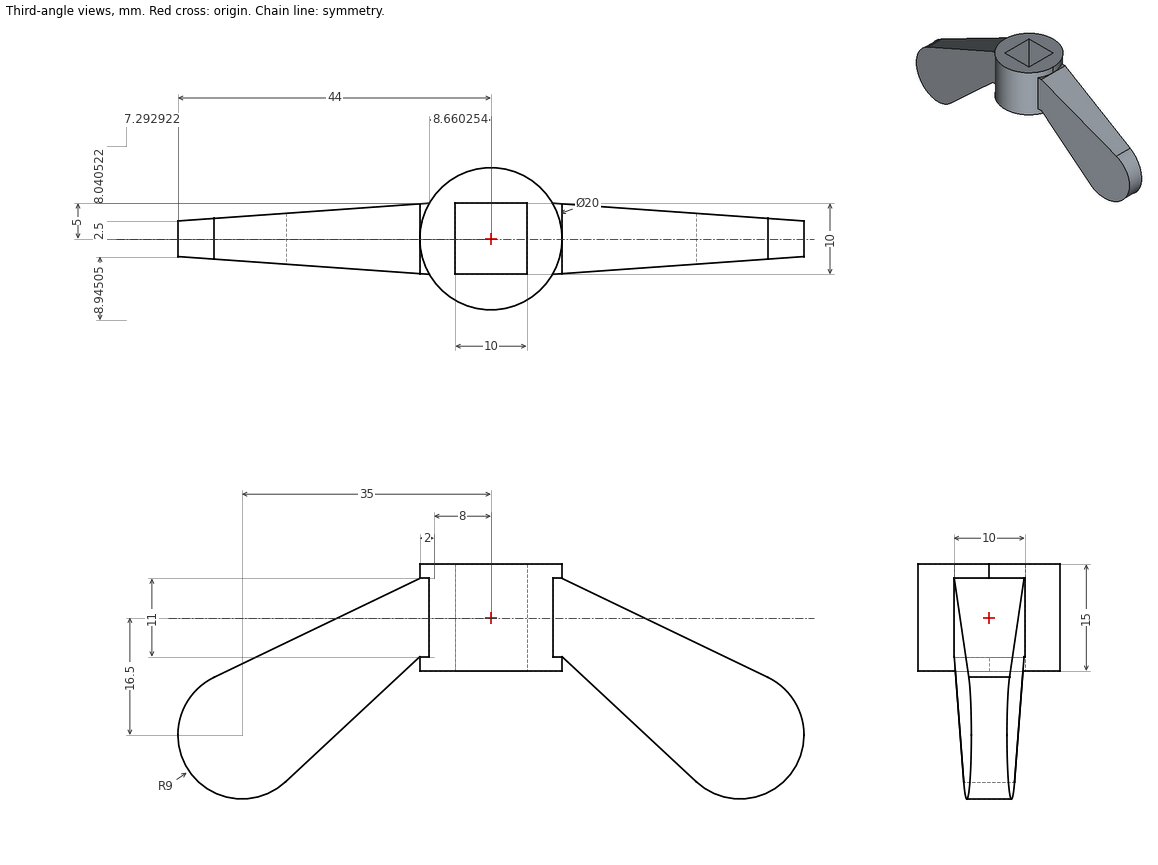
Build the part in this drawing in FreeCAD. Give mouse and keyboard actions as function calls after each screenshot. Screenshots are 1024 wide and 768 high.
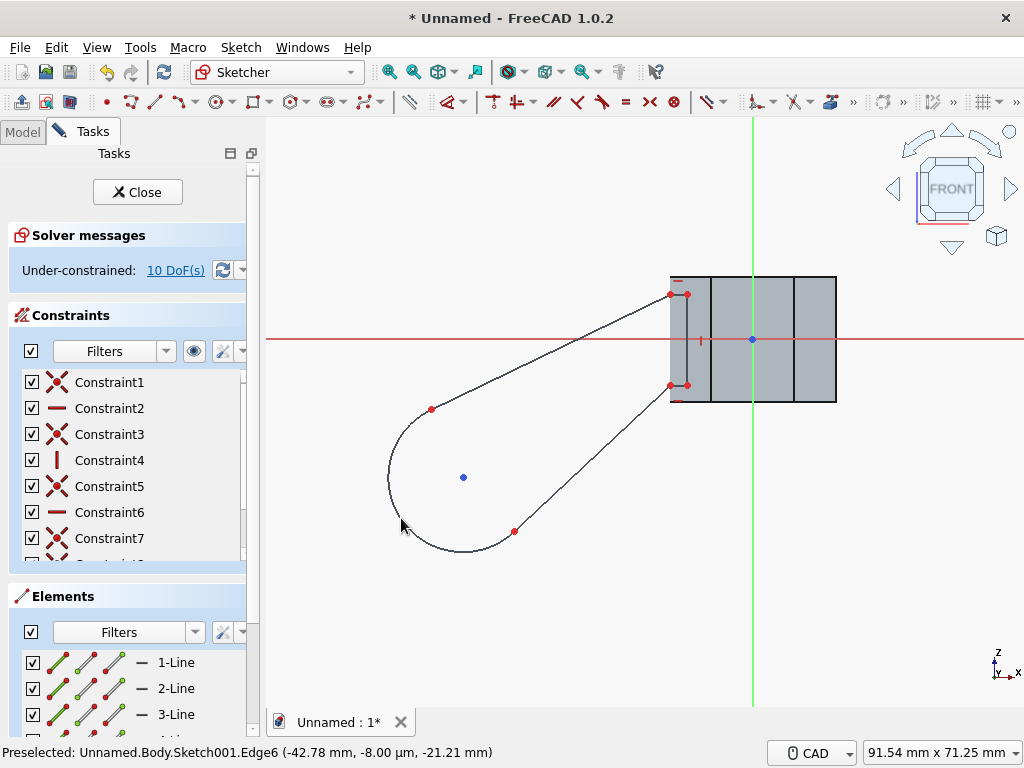
click(503, 375)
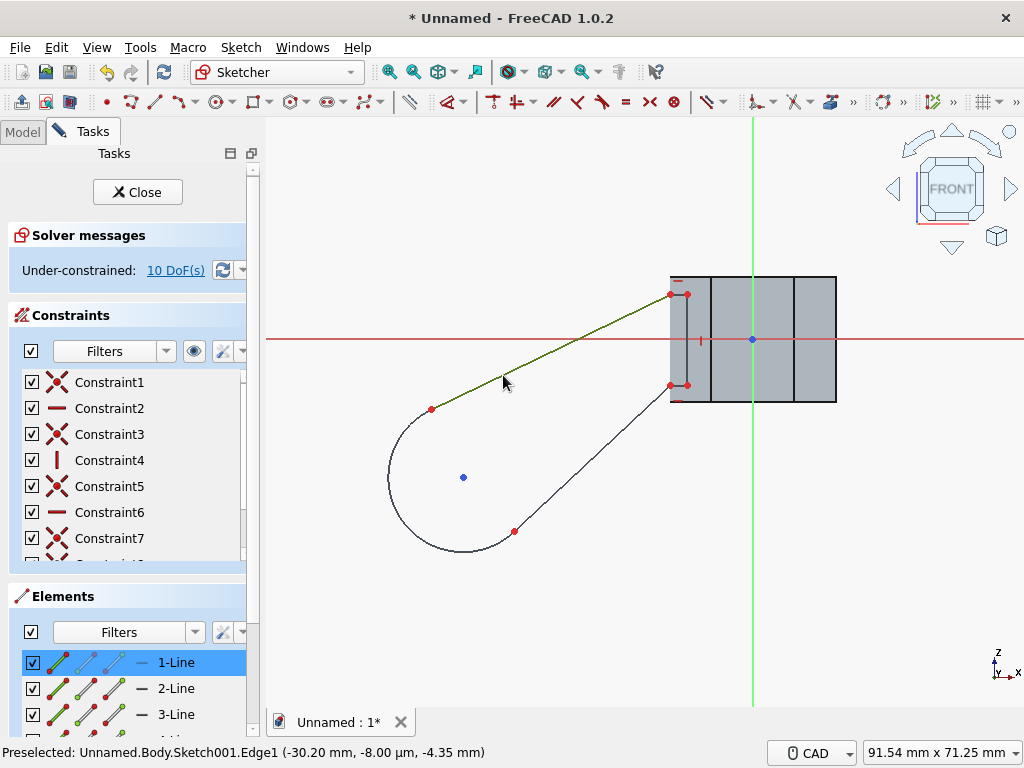
click(389, 471)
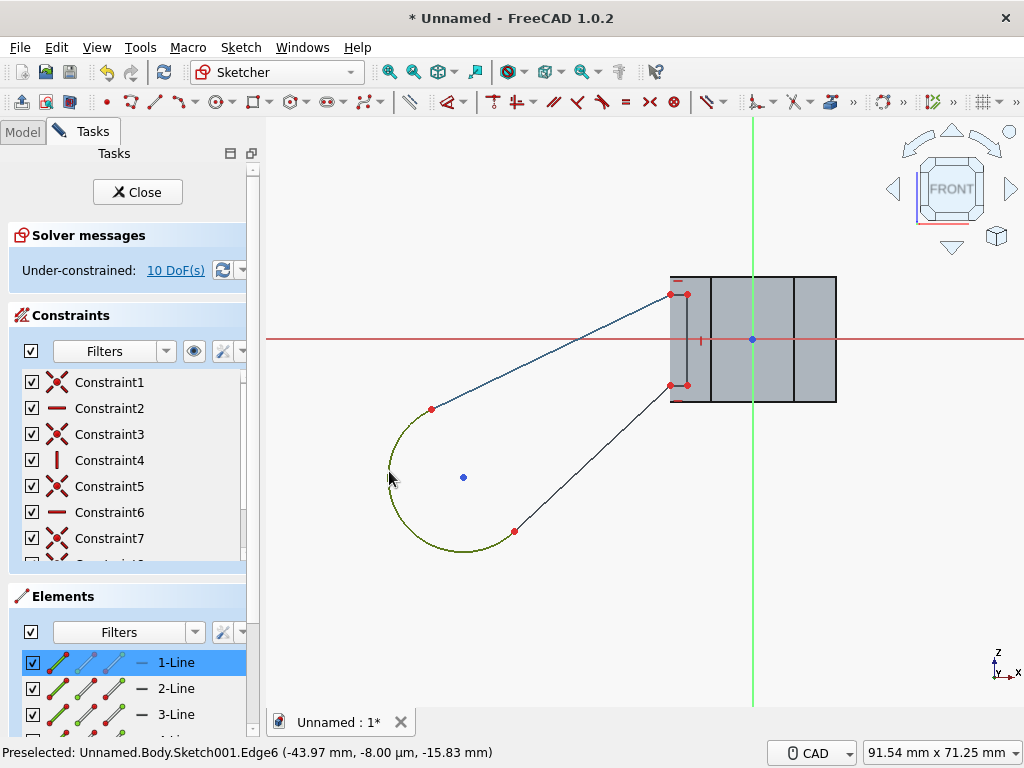
click(602, 102)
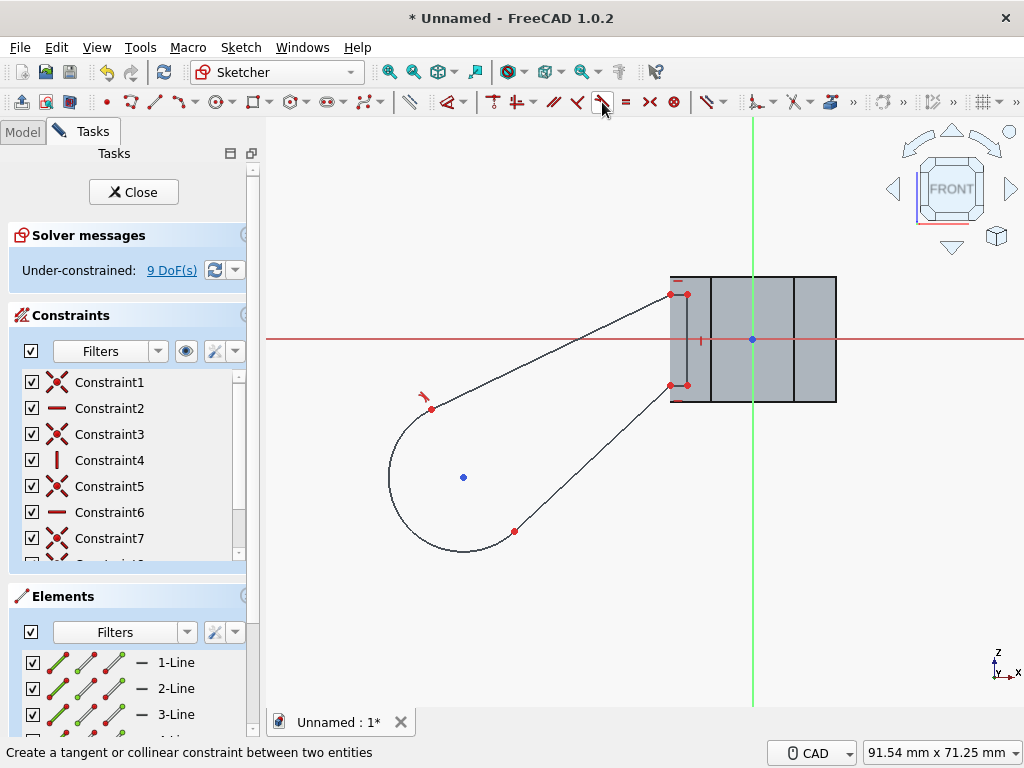
click(623, 430)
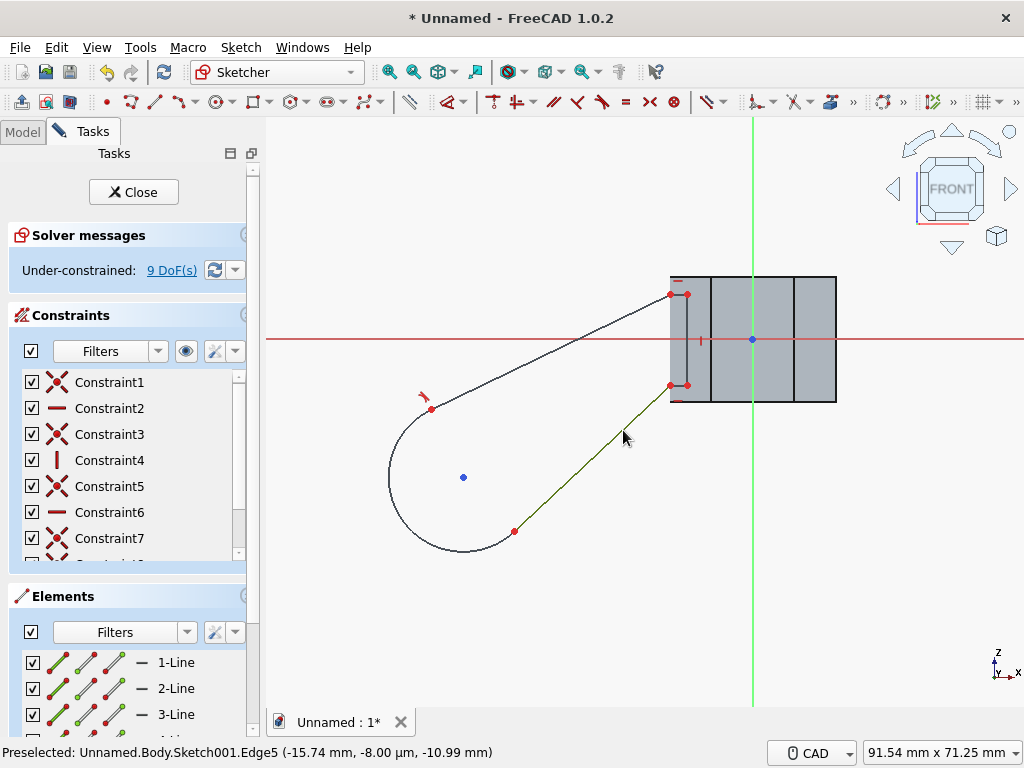
click(389, 470)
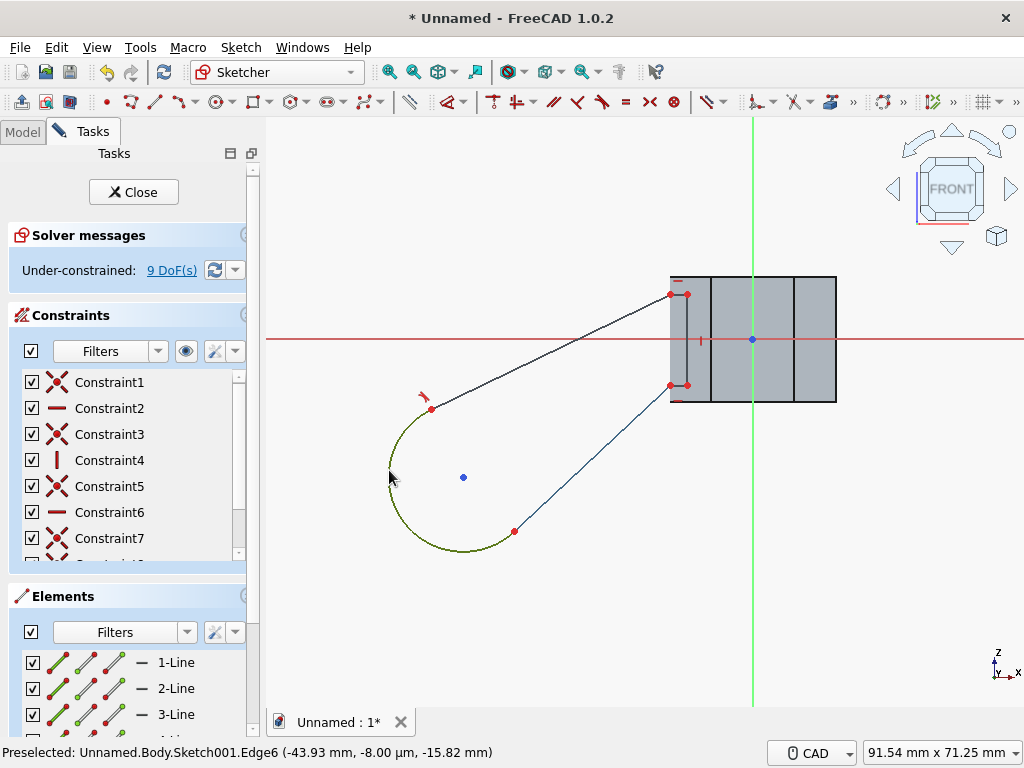
key(t)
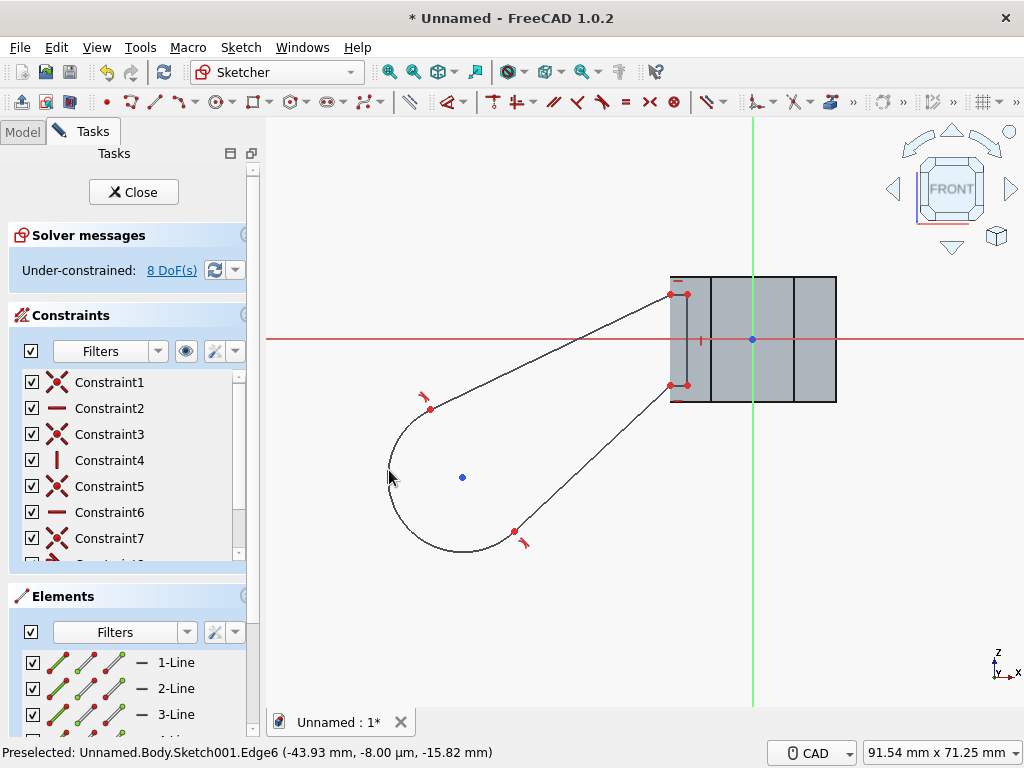
click(670, 295)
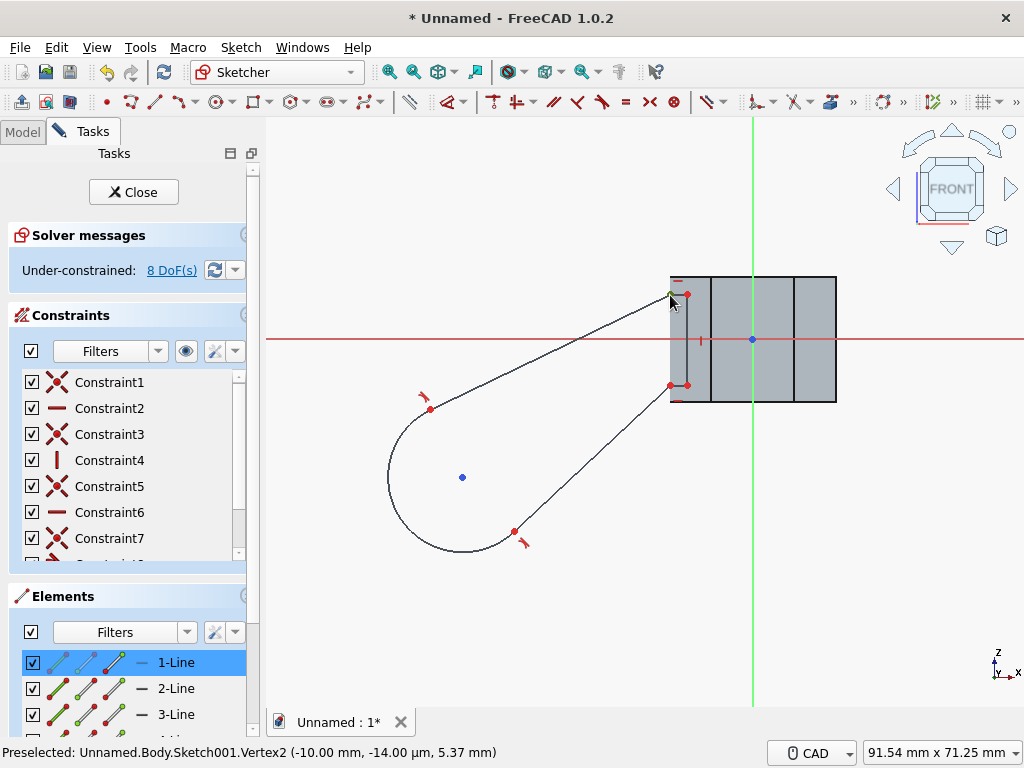
click(670, 386)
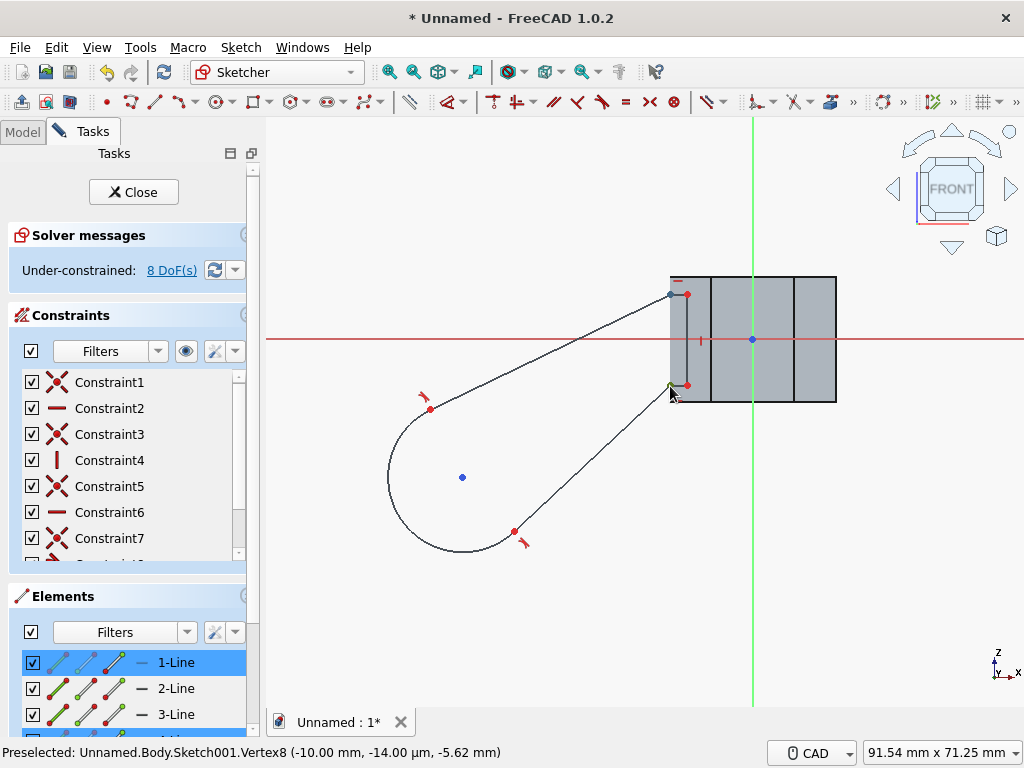
click(334, 339)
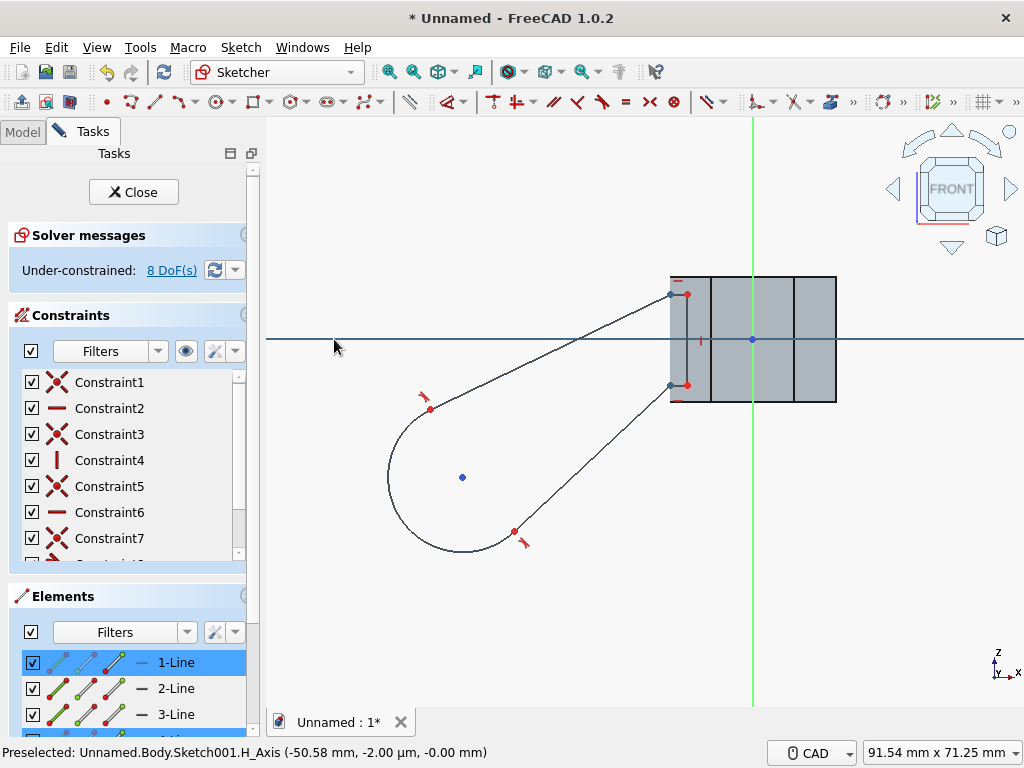
click(650, 102)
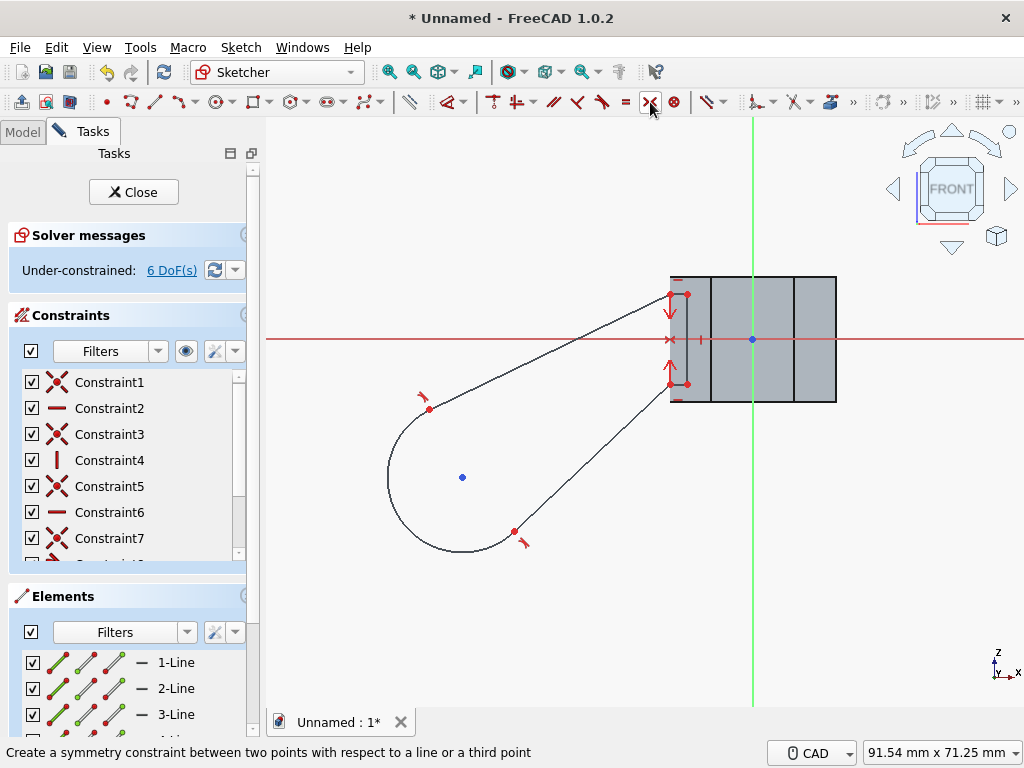
click(448, 102)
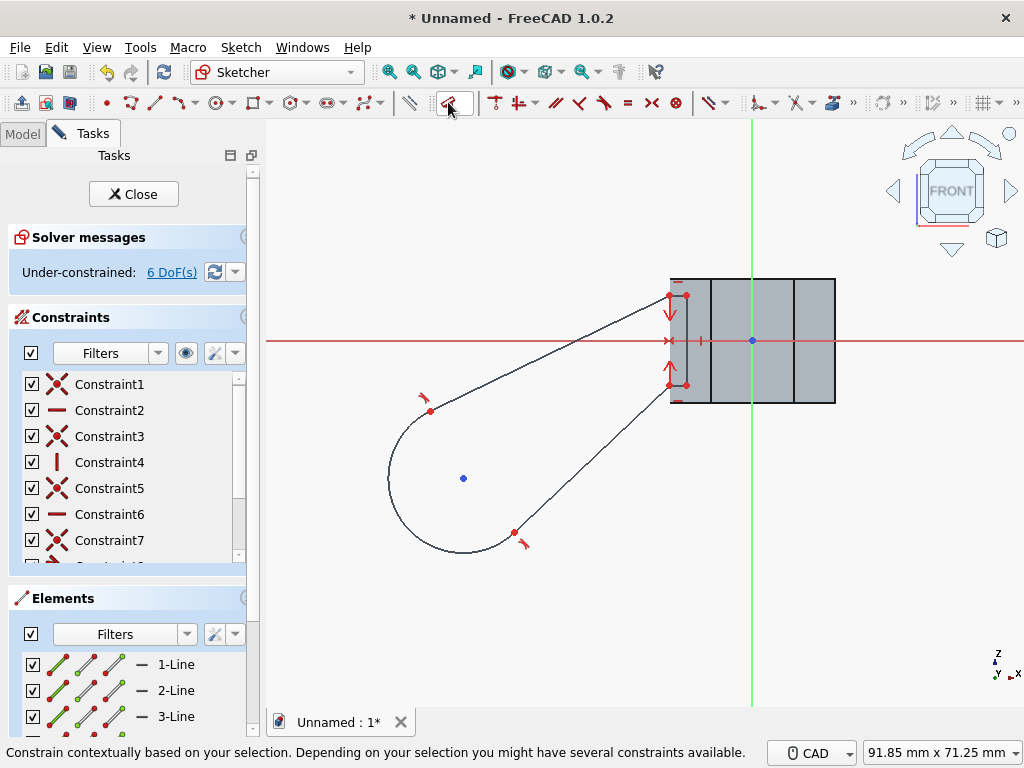
click(389, 472)
click(357, 469)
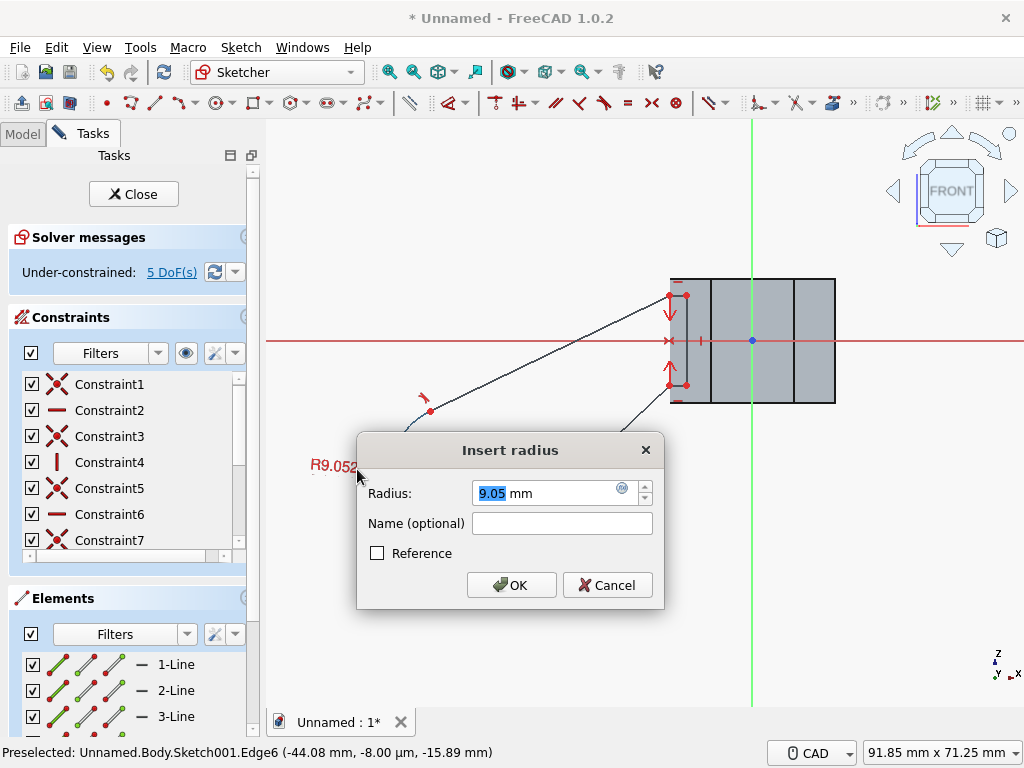
text(9)
key(Return)